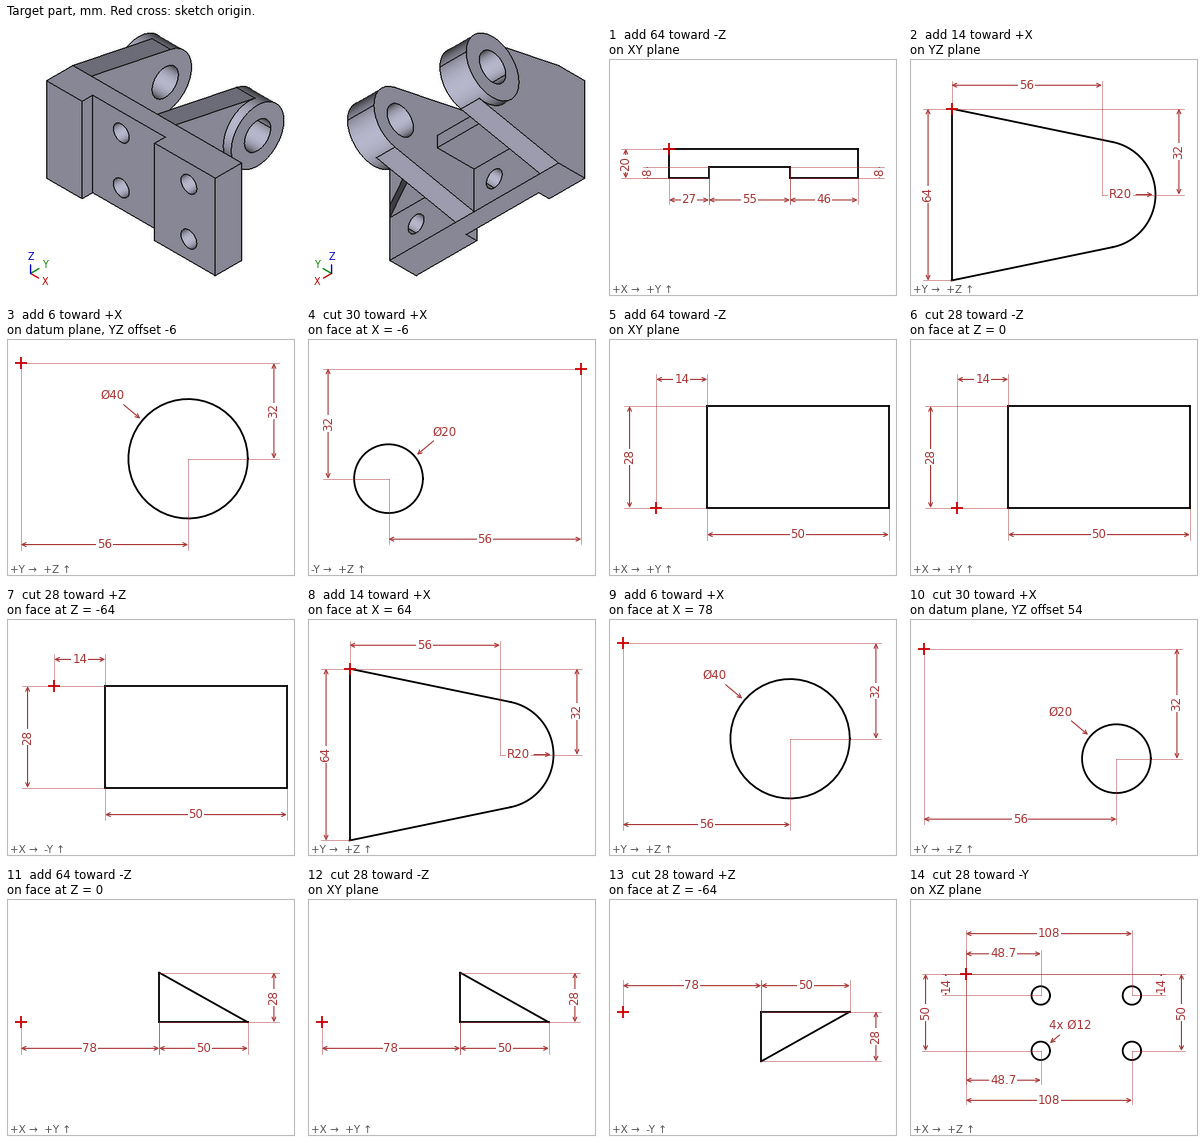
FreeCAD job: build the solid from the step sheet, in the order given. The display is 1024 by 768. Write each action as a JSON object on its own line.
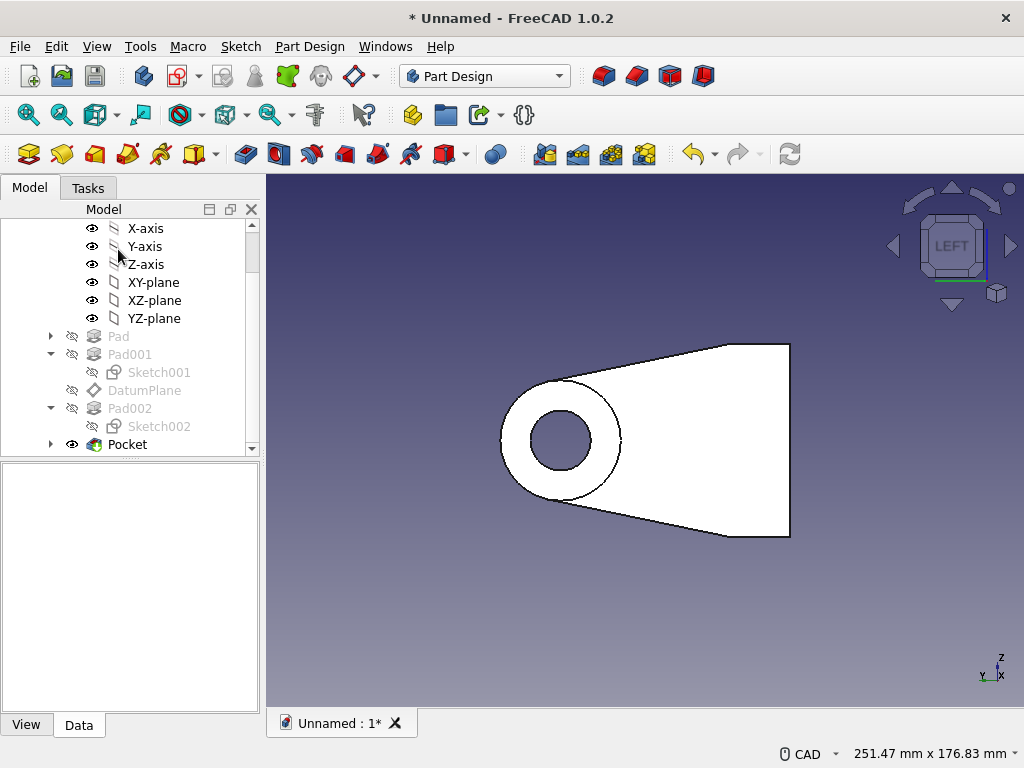
{"action": "left_click", "coordinate": [29, 116]}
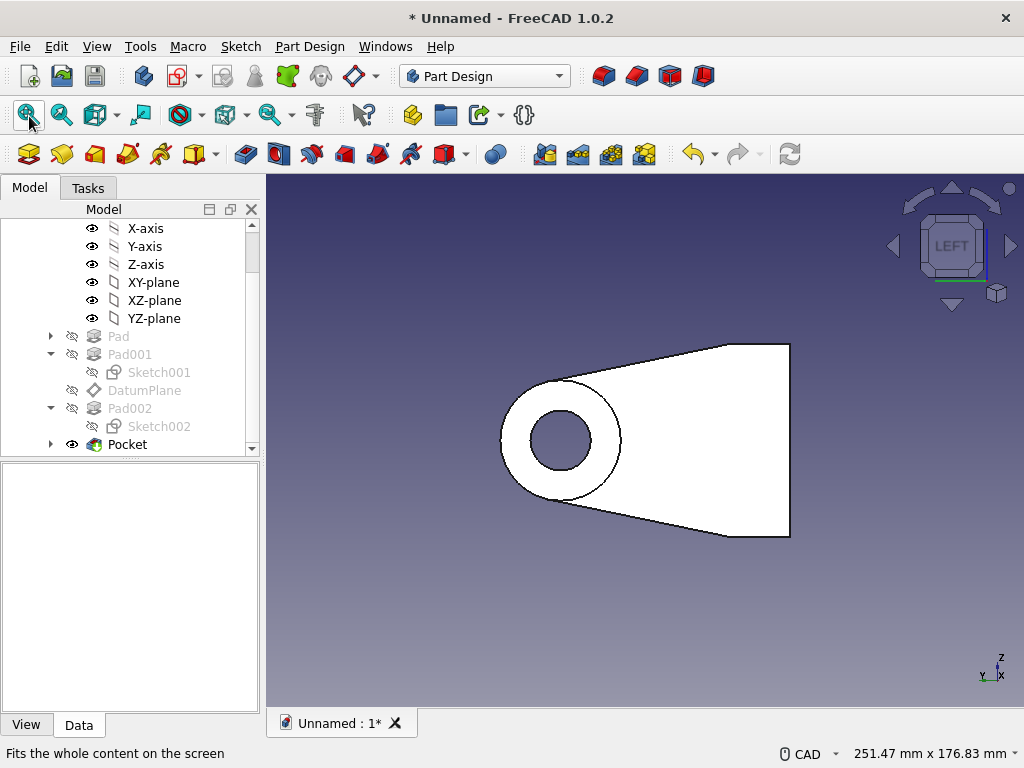
{"action": "left_click", "coordinate": [176, 76]}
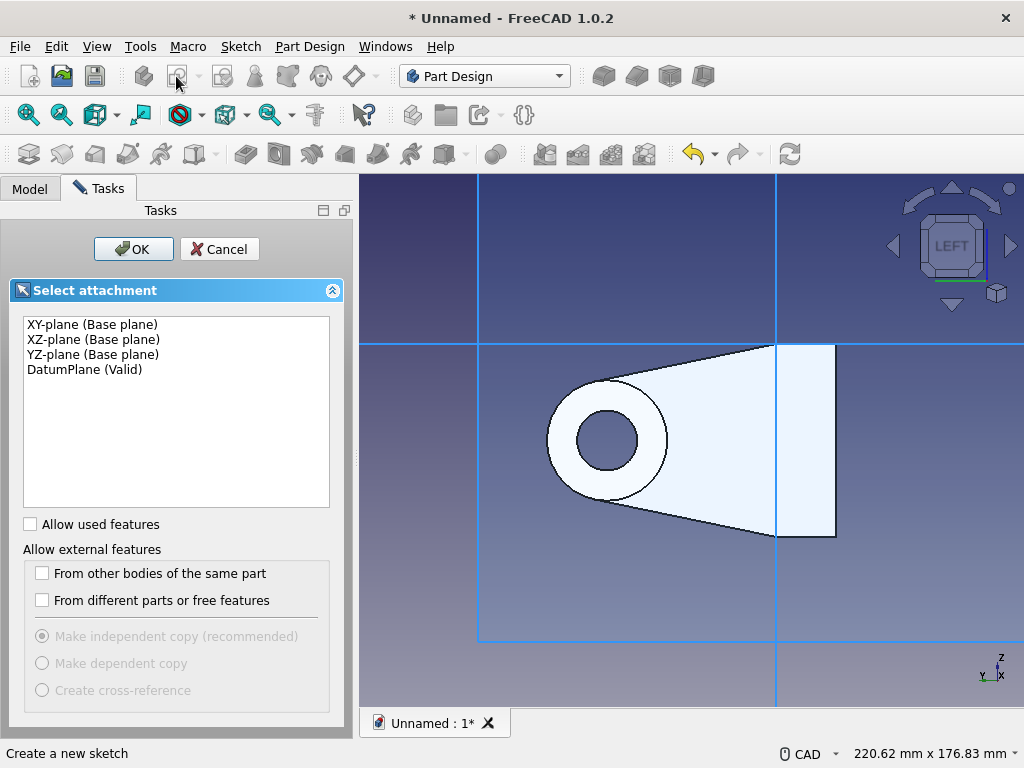
{"action": "left_click", "coordinate": [84, 324]}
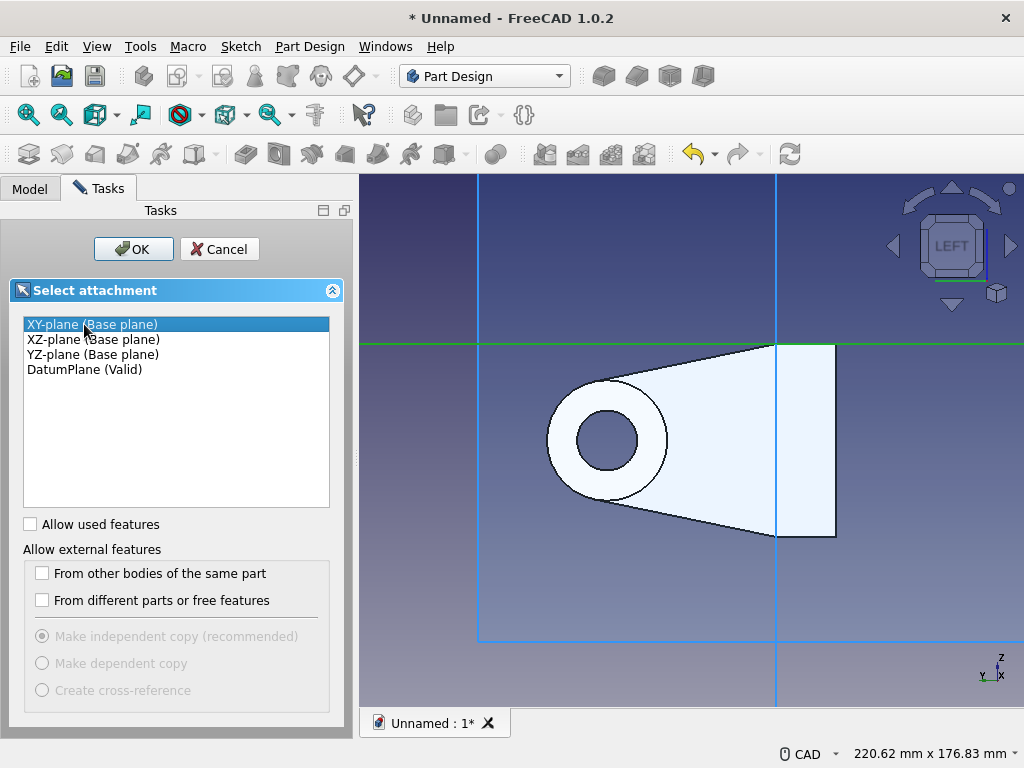
{"action": "left_click", "coordinate": [134, 249]}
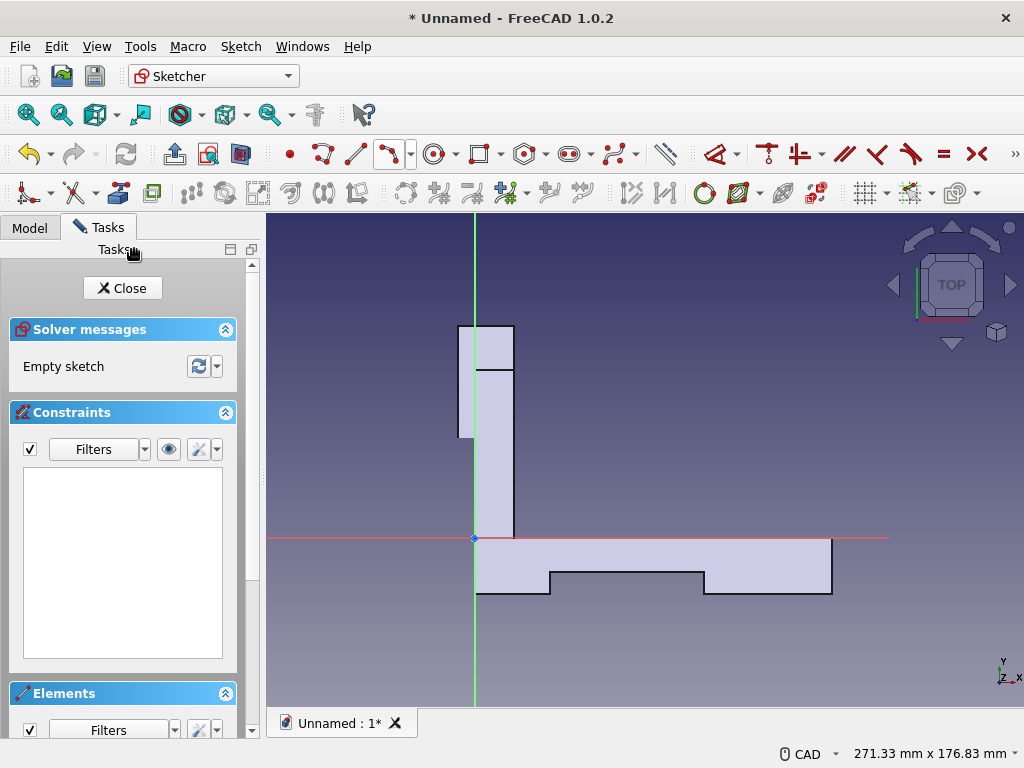
{"action": "scroll", "coordinate": [554, 531], "scroll_direction": "up", "scroll_amount": 4}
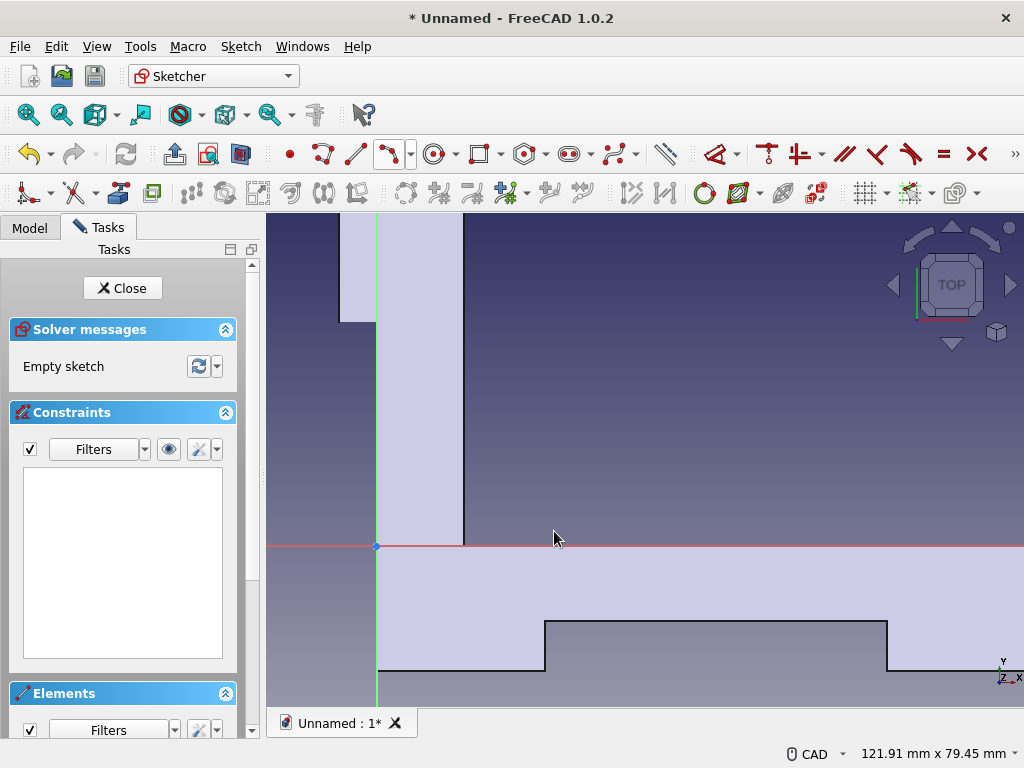
{"action": "left_click", "coordinate": [478, 154]}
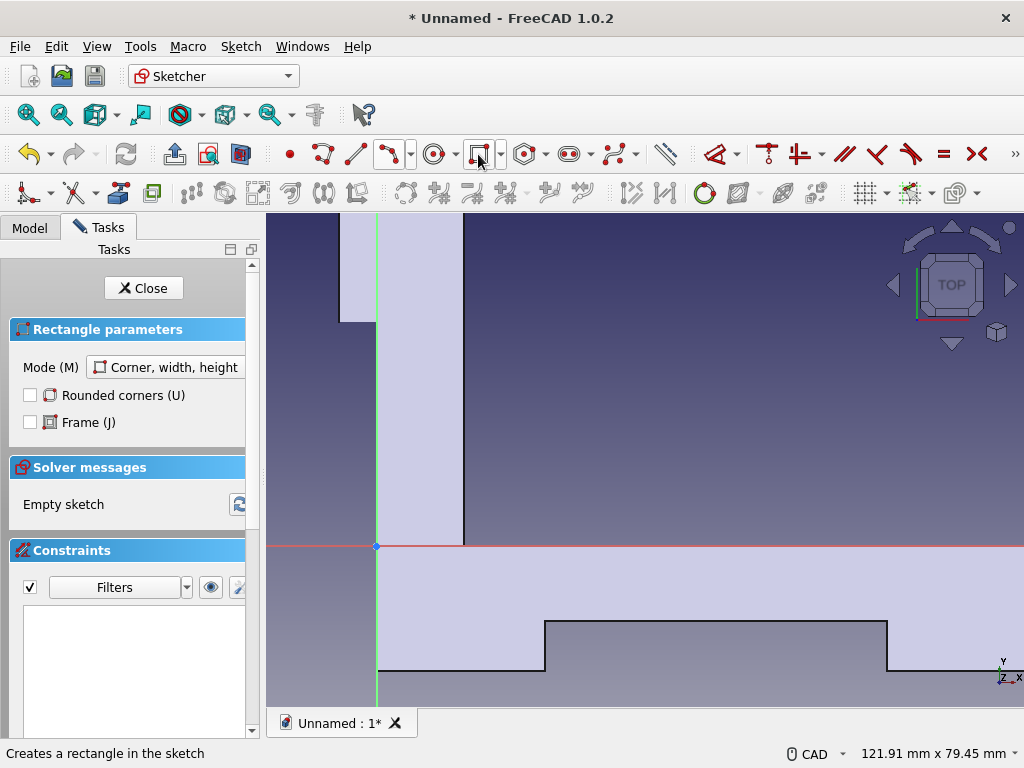
{"action": "left_click", "coordinate": [464, 372]}
{"action": "left_click", "coordinate": [775, 546]}
{"action": "key", "text": "Escape"}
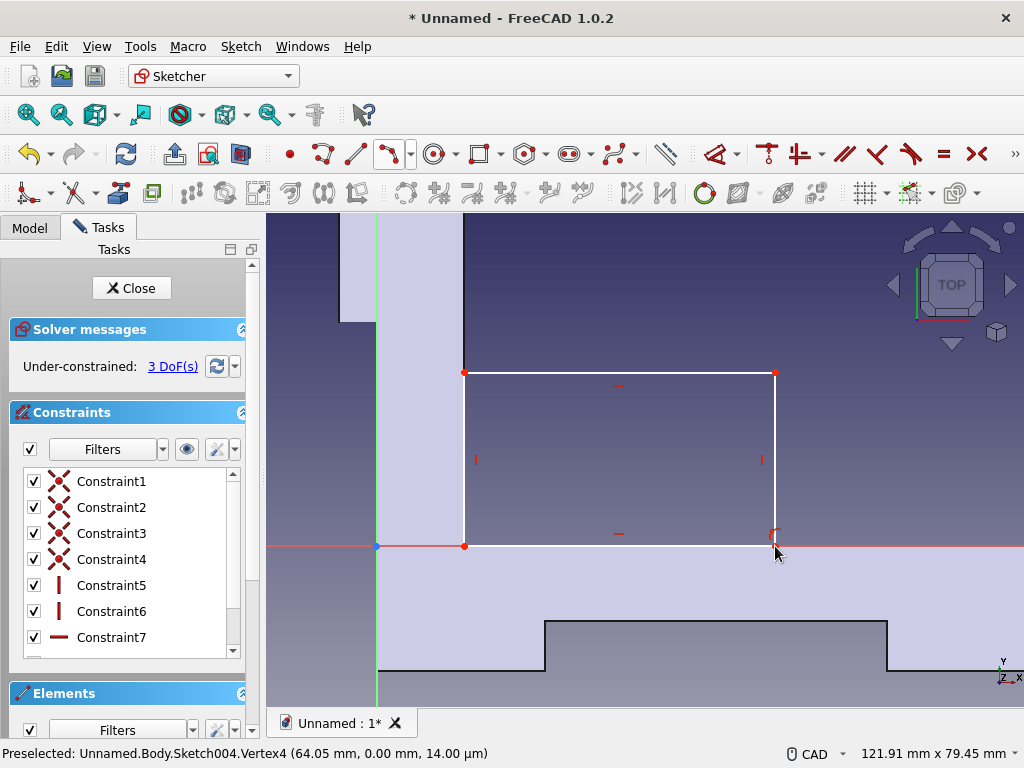
{"action": "left_click", "coordinate": [714, 154]}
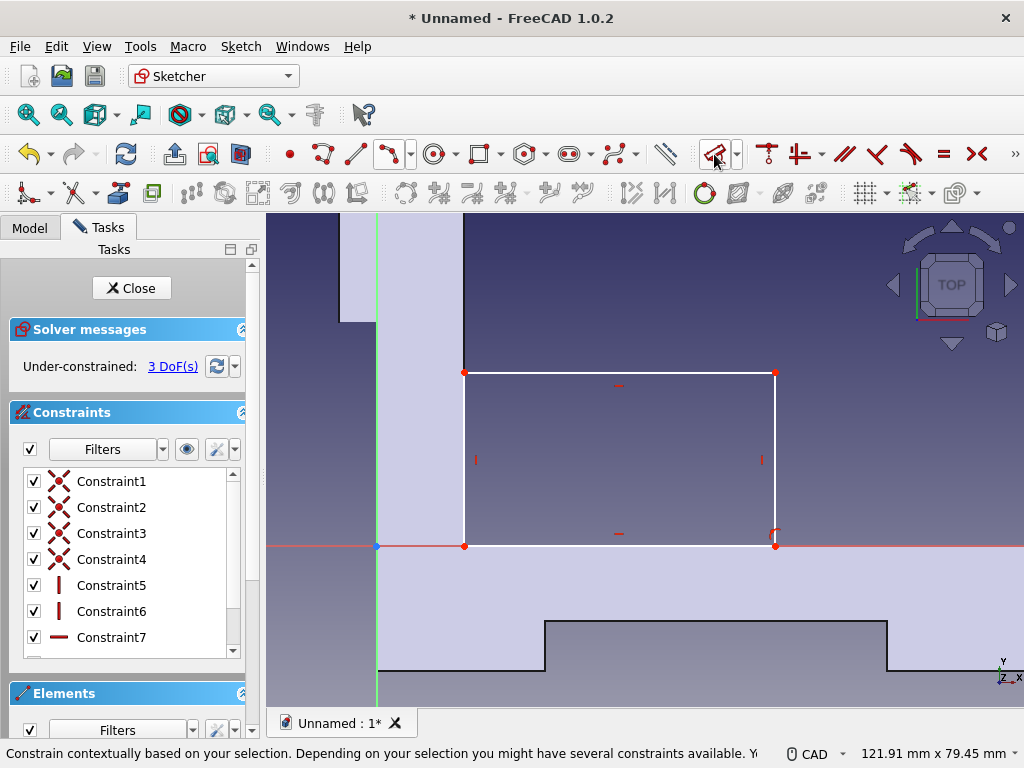
{"action": "left_click", "coordinate": [464, 425]}
{"action": "left_click", "coordinate": [430, 460]}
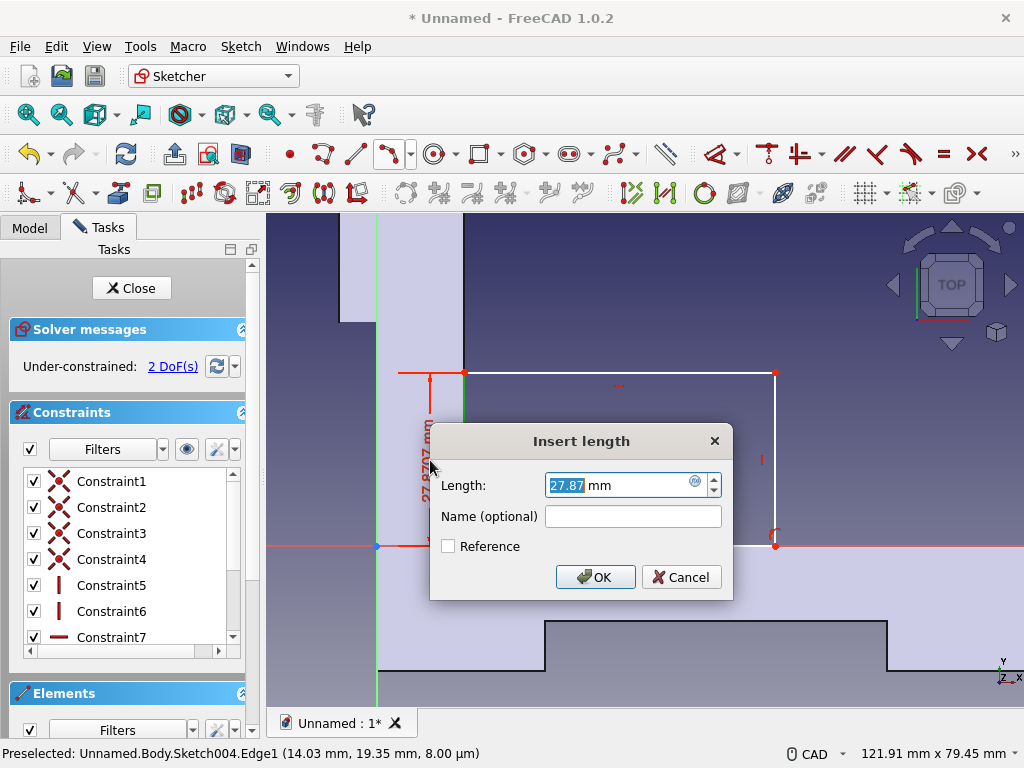
{"action": "type", "text": "28"}
{"action": "key", "text": "Return"}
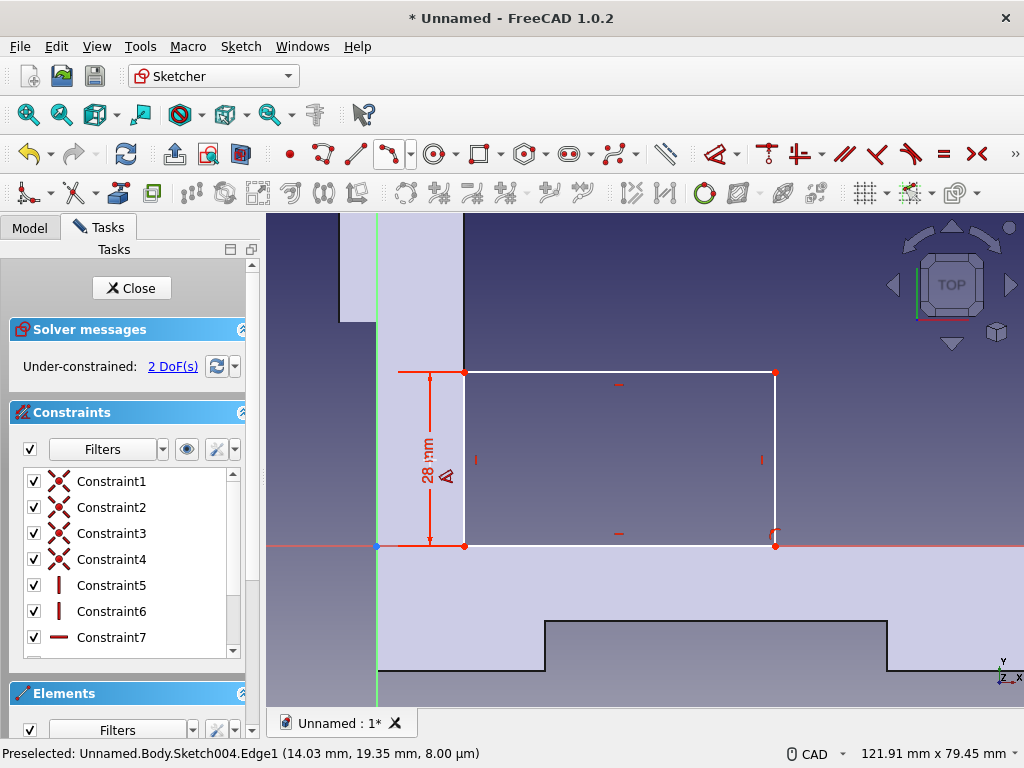
{"action": "left_click", "coordinate": [557, 546]}
{"action": "left_click", "coordinate": [620, 580]}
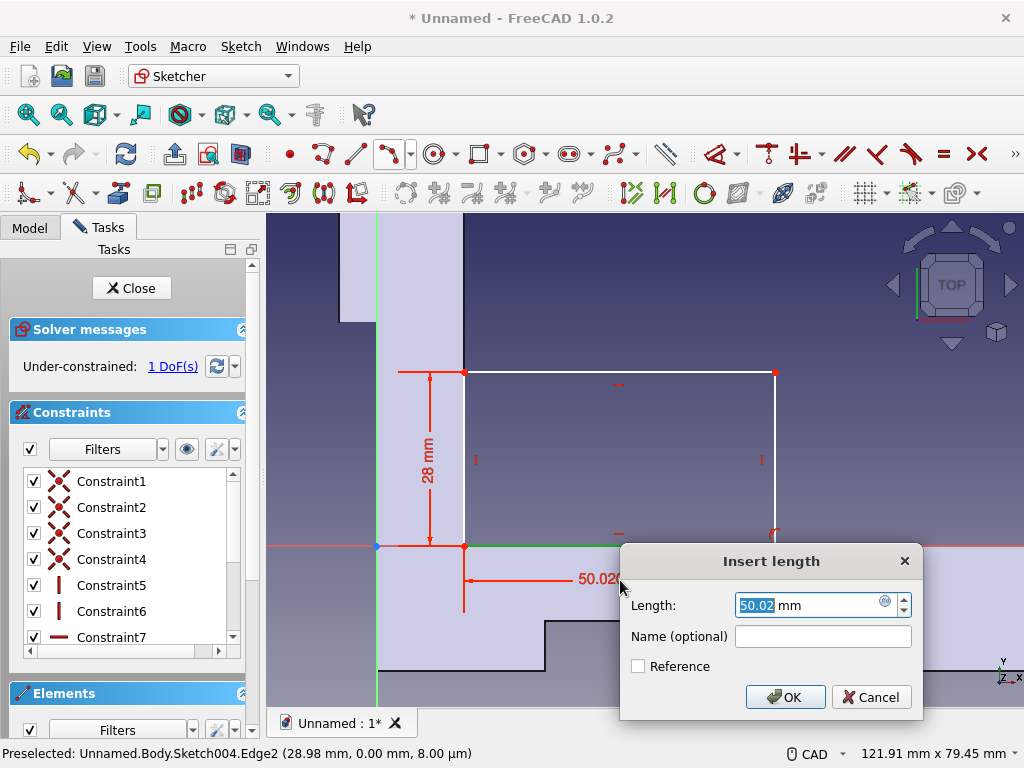
{"action": "type", "text": "50"}
{"action": "key", "text": "Return"}